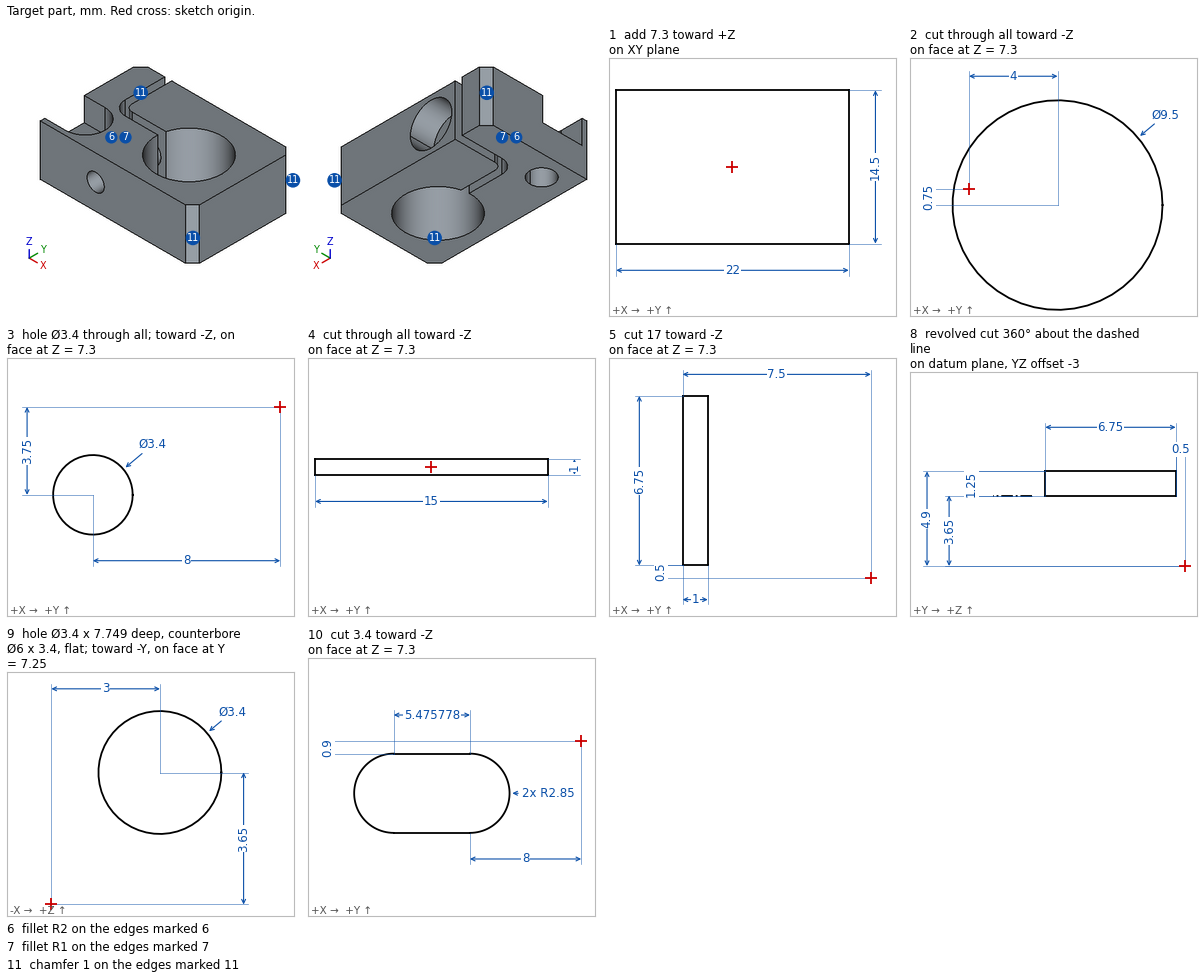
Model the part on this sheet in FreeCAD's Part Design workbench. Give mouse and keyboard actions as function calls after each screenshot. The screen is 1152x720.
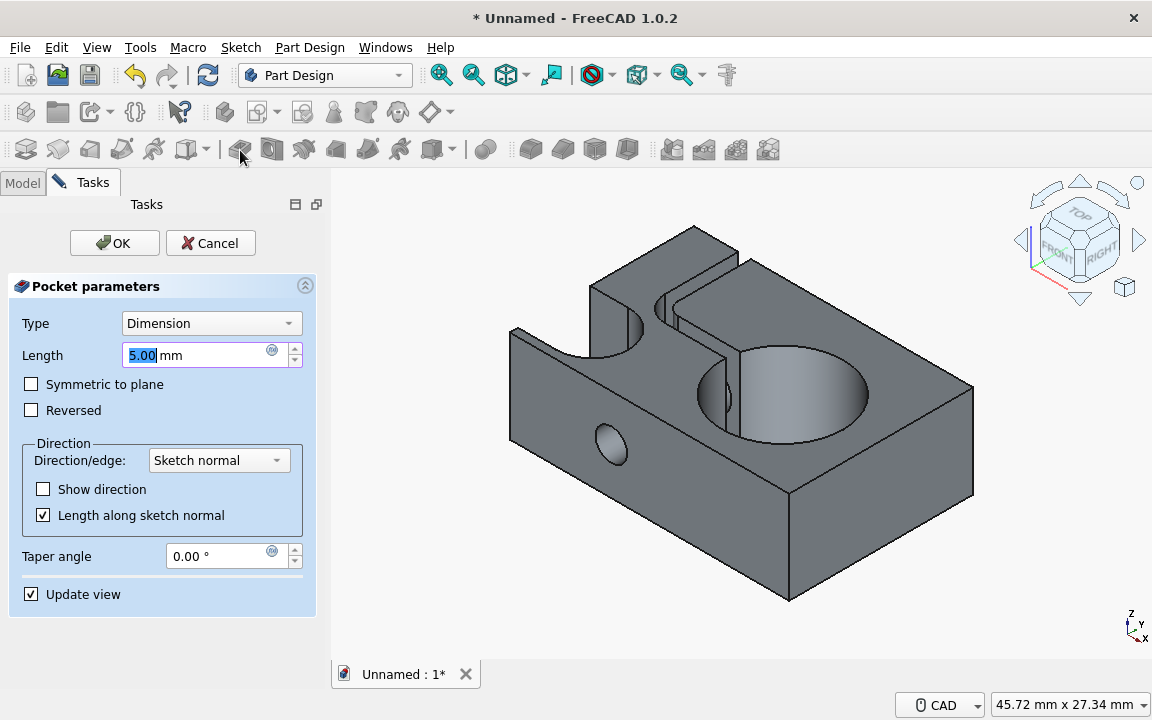
text(3.4)
key(Tab)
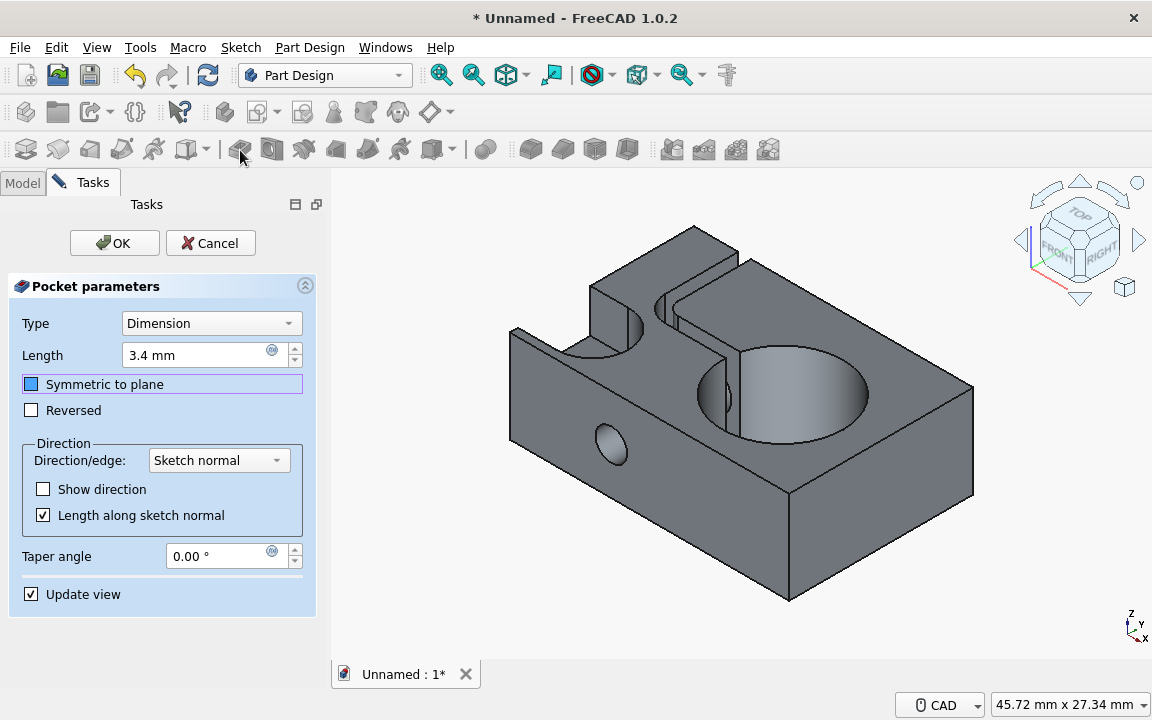
click(115, 243)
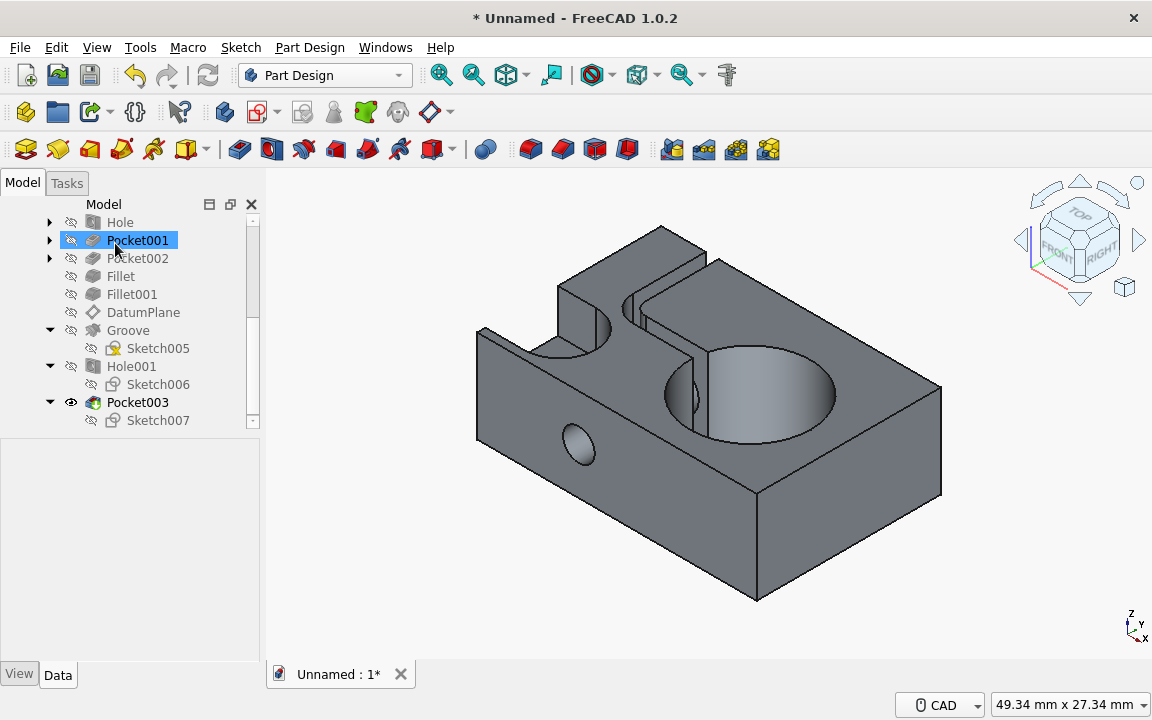
click(757, 546)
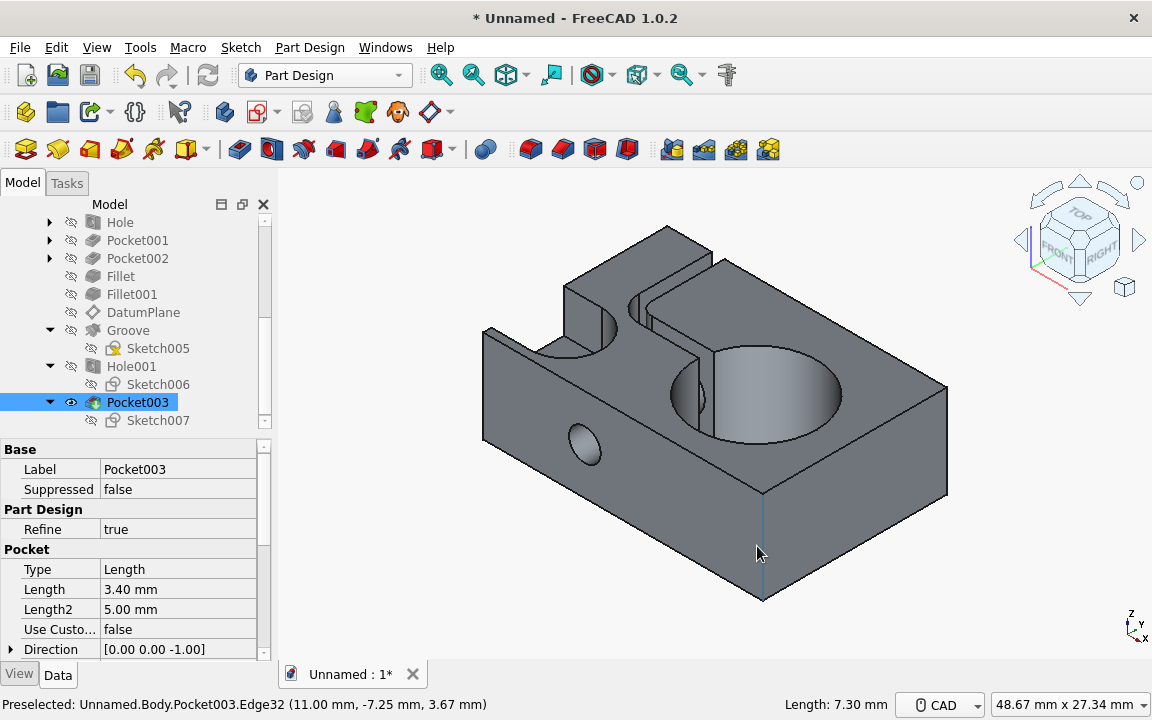
key(2)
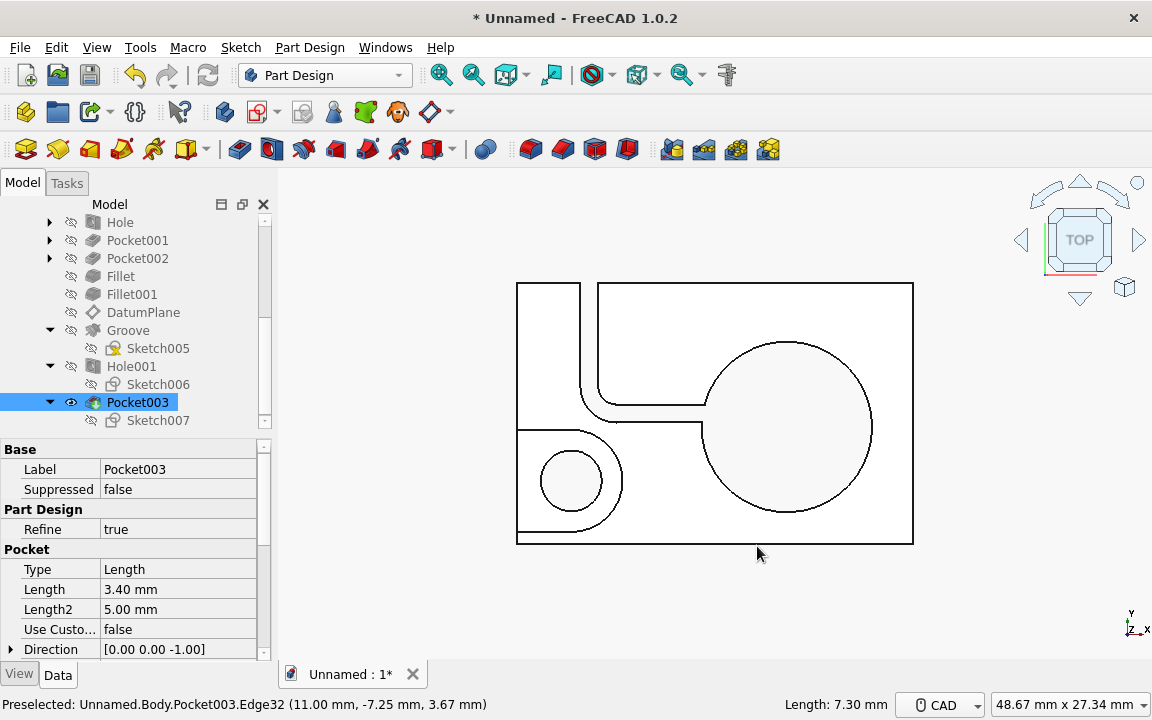
key(0)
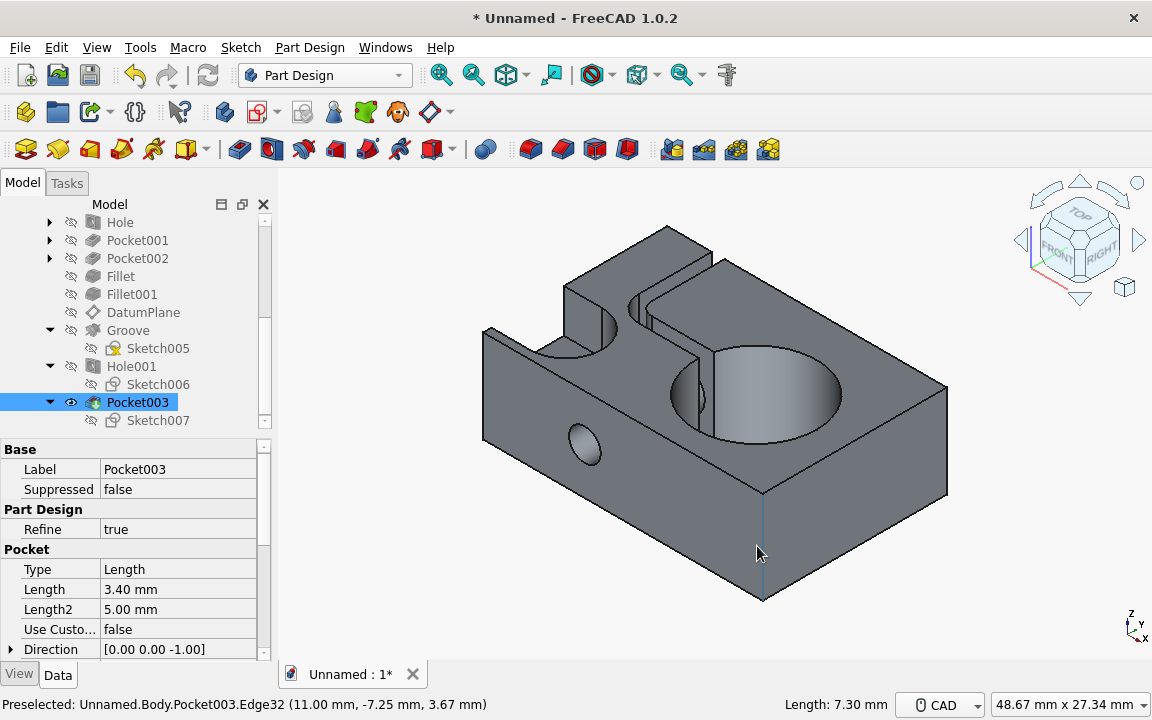
key(1)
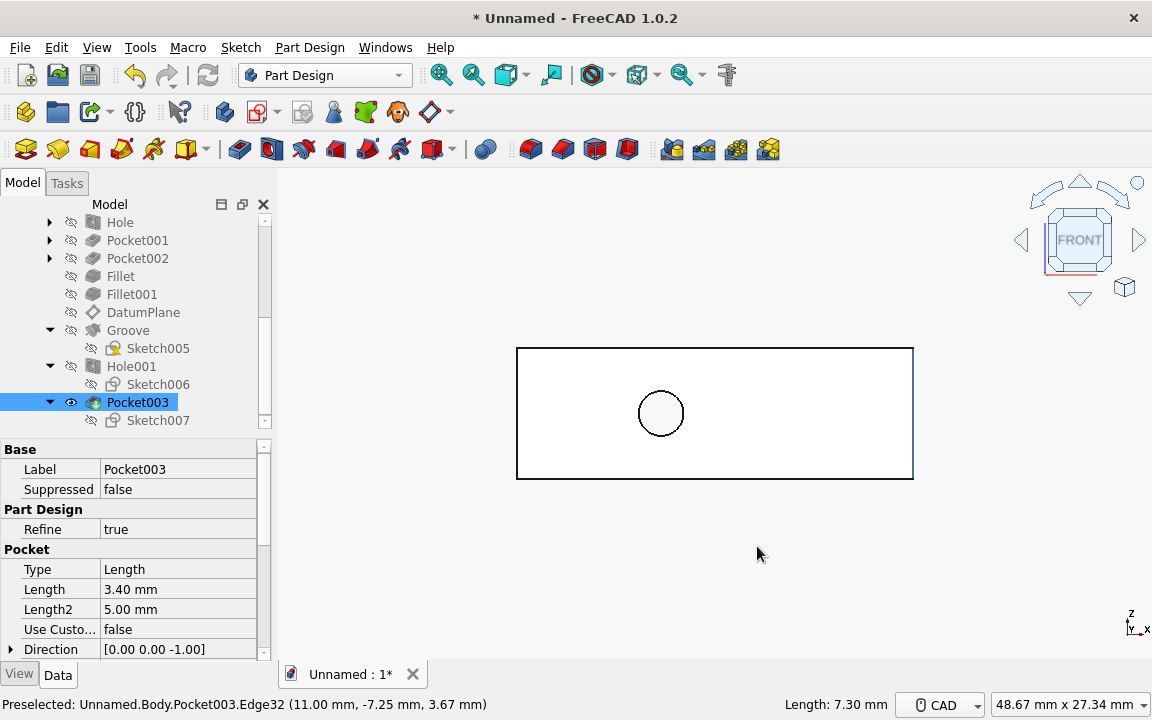
key(3)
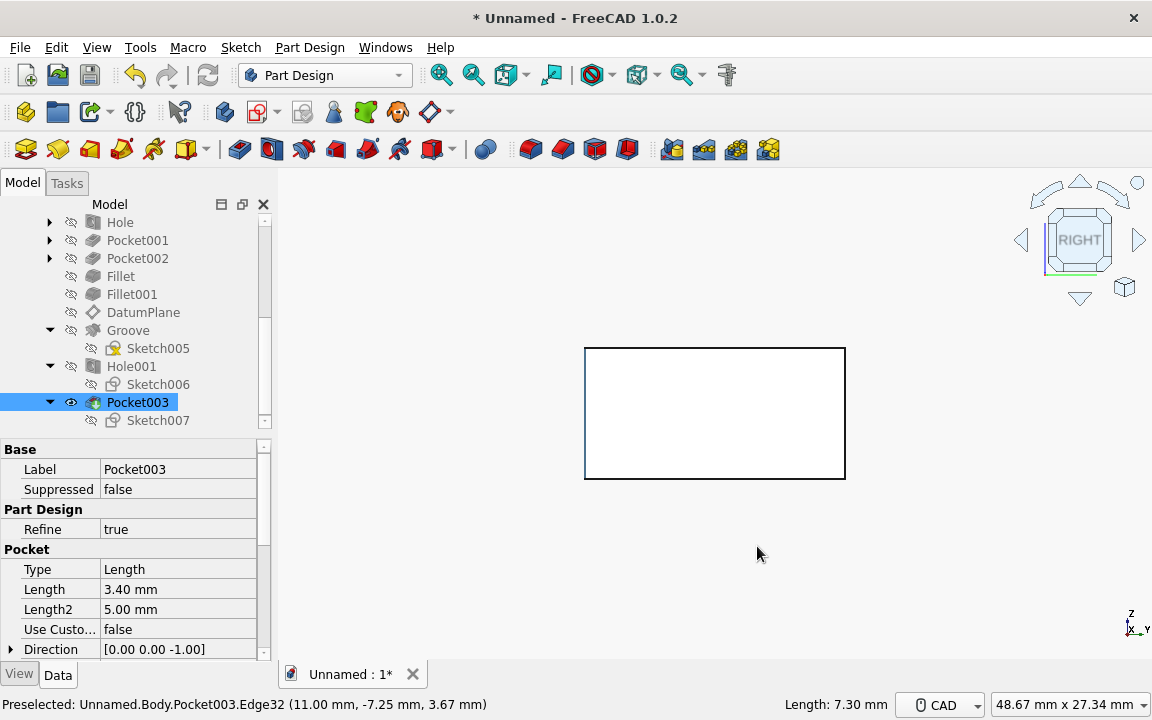
click(442, 76)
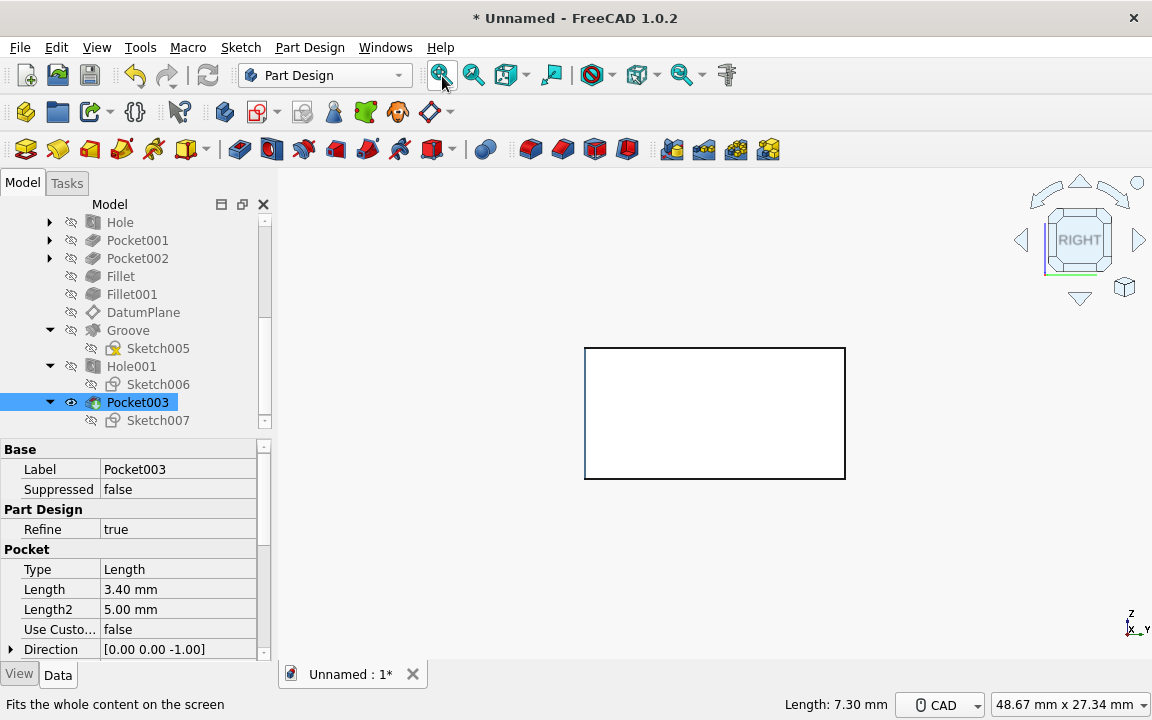
click(845, 412, ctrl)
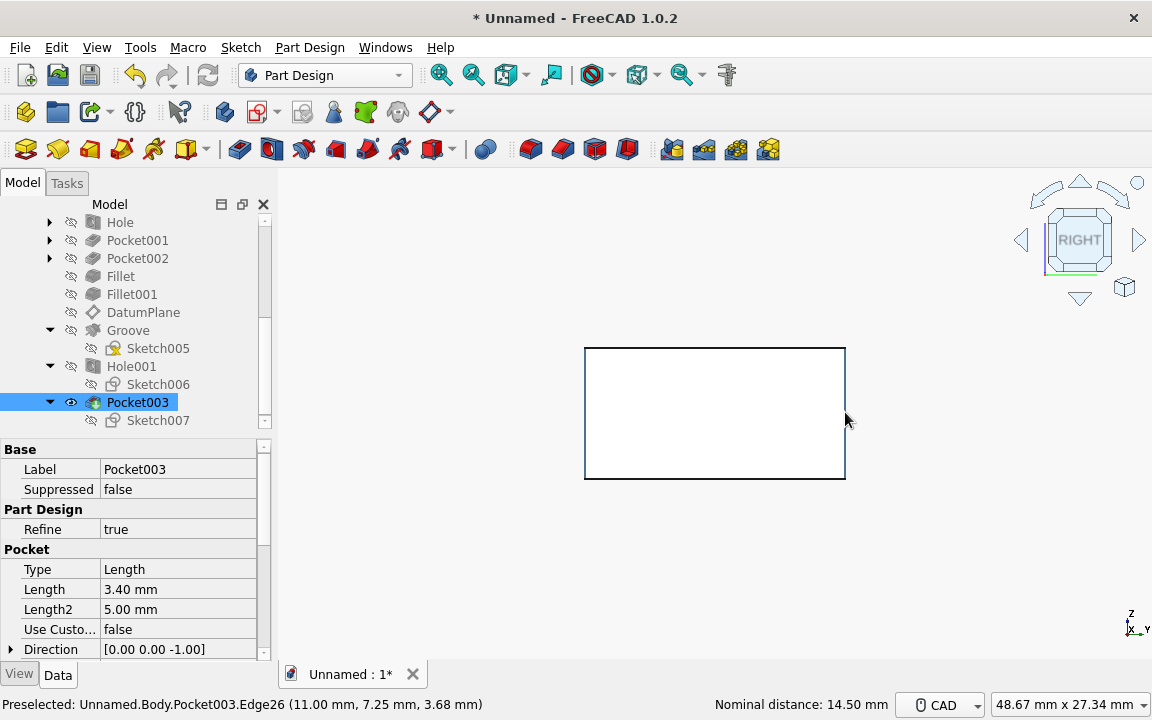
key(5)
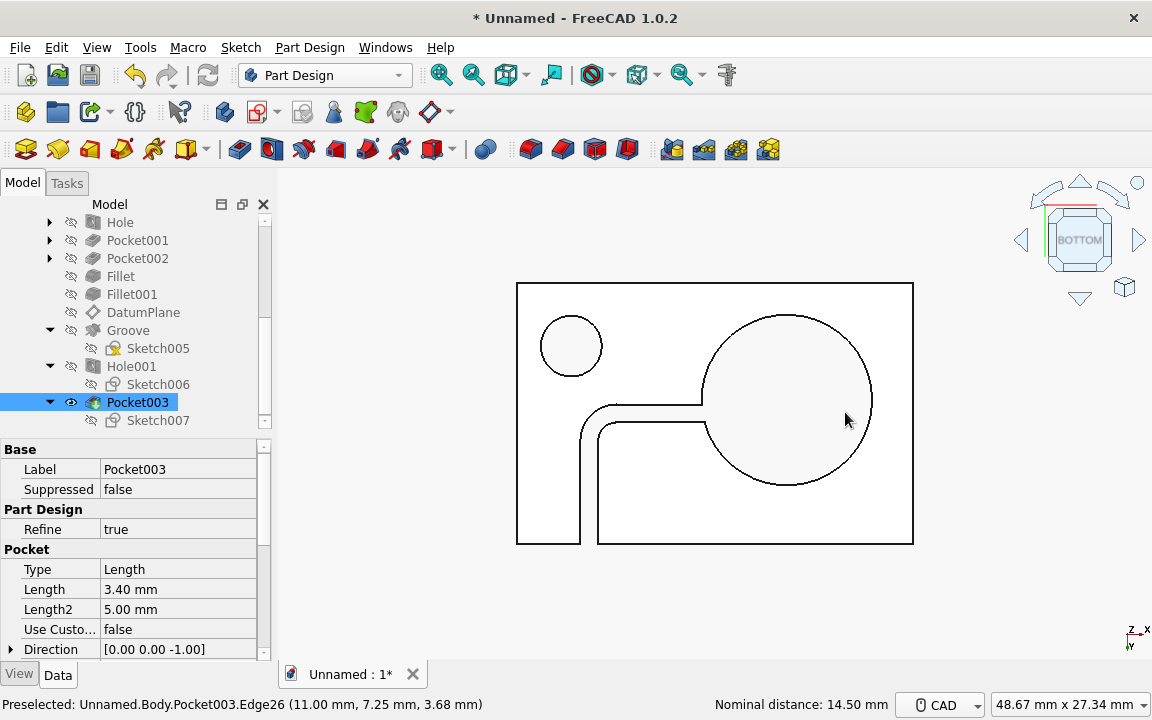
key(4)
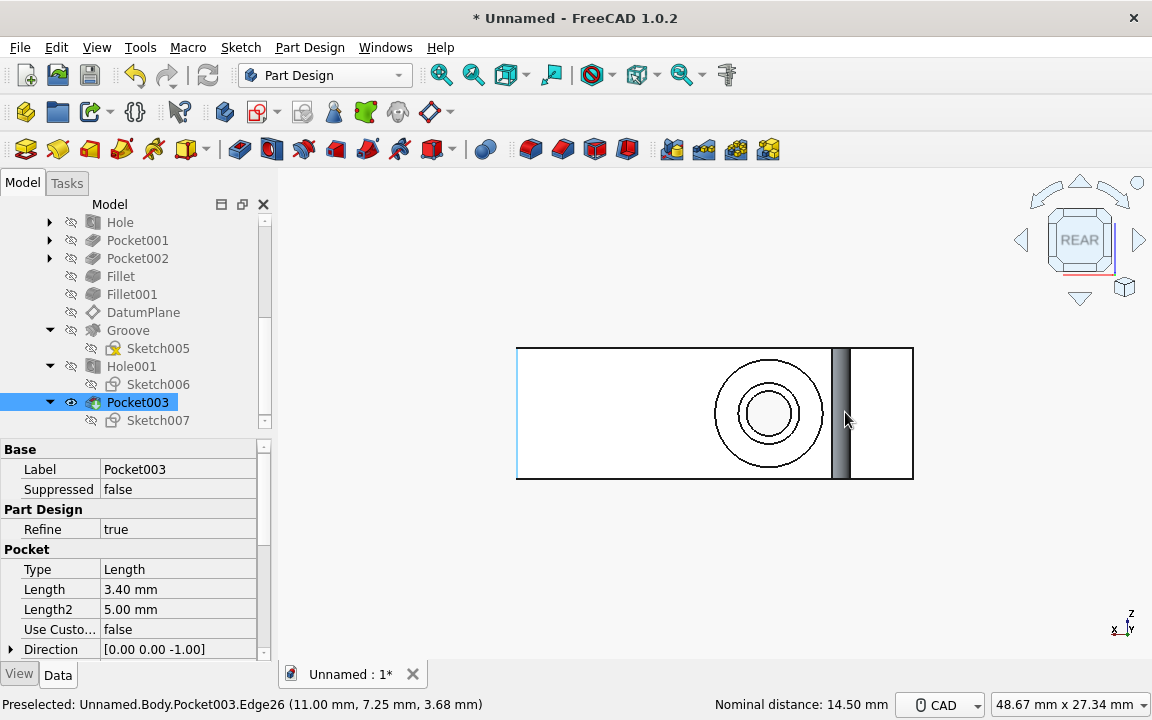
click(913, 413, ctrl)